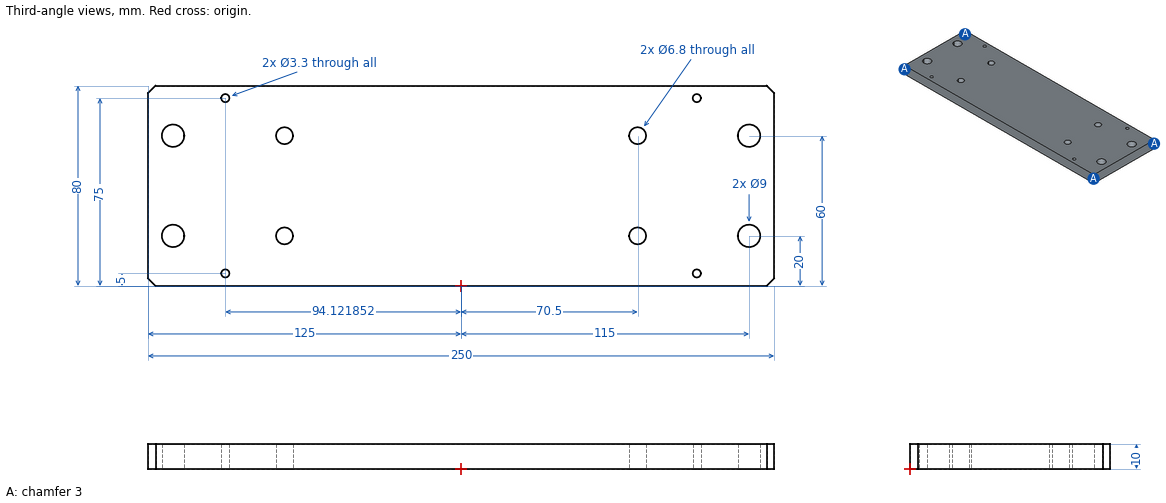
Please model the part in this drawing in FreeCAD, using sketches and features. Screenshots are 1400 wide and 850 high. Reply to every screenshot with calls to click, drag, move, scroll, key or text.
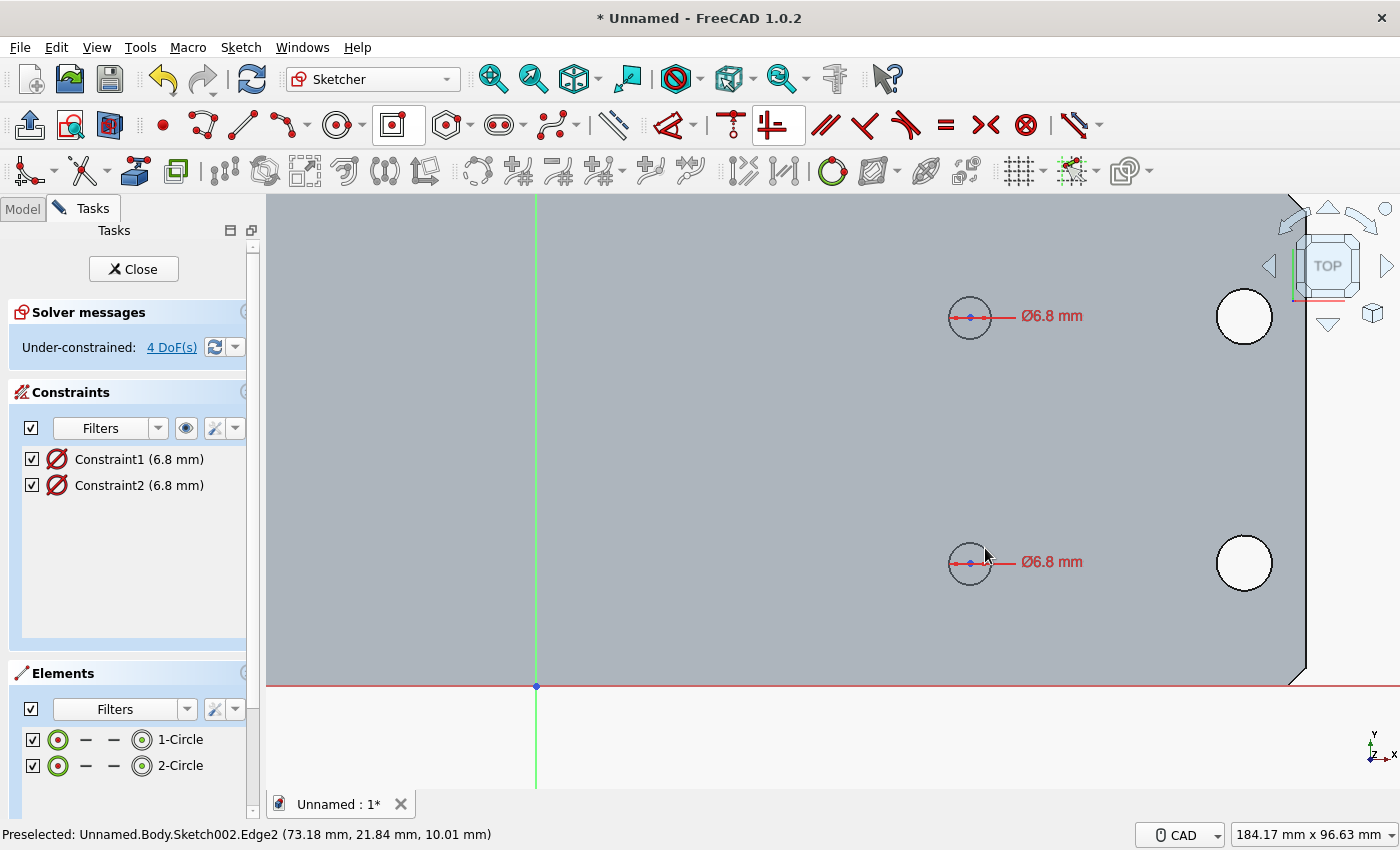
click(970, 318)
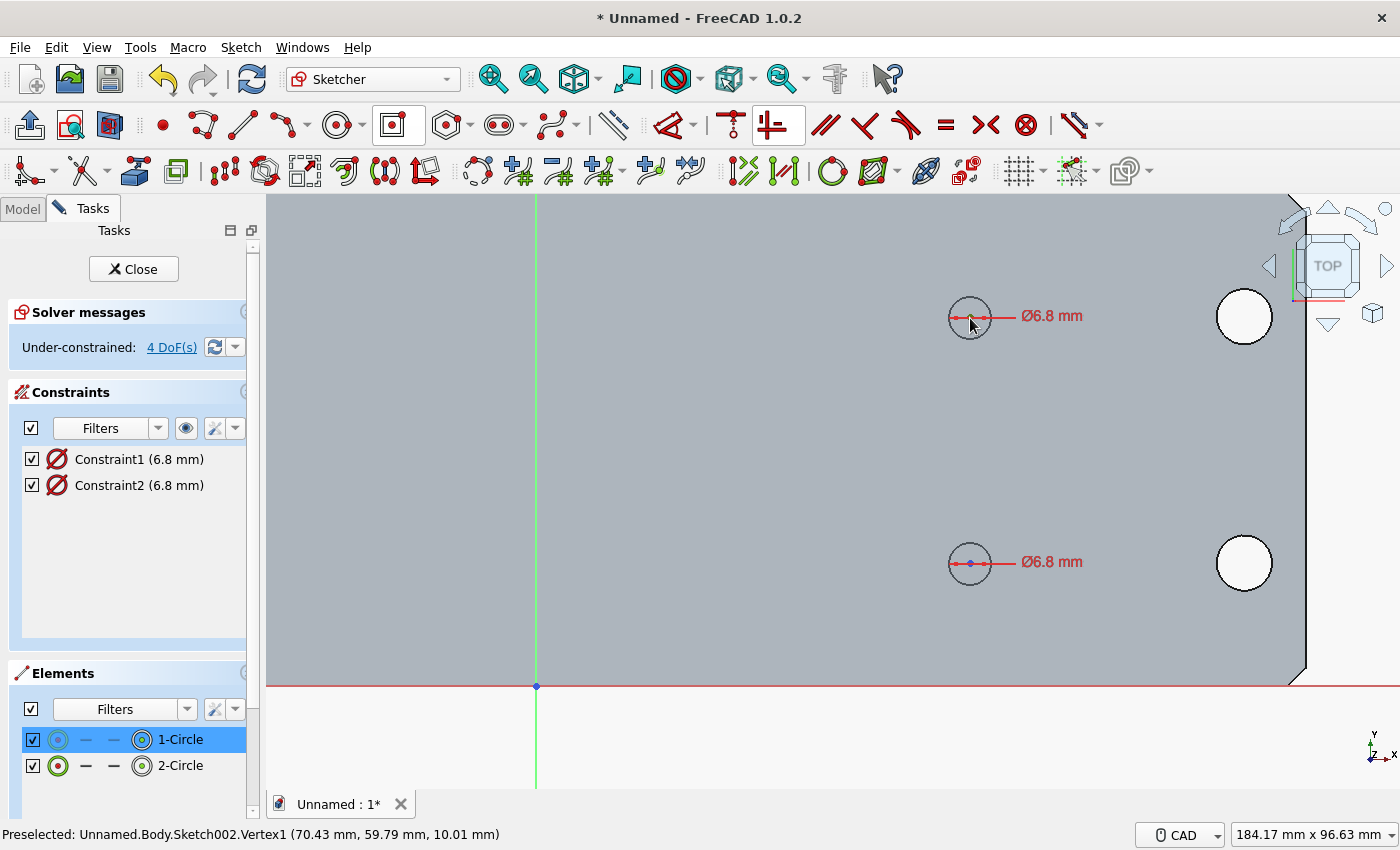
click(970, 564)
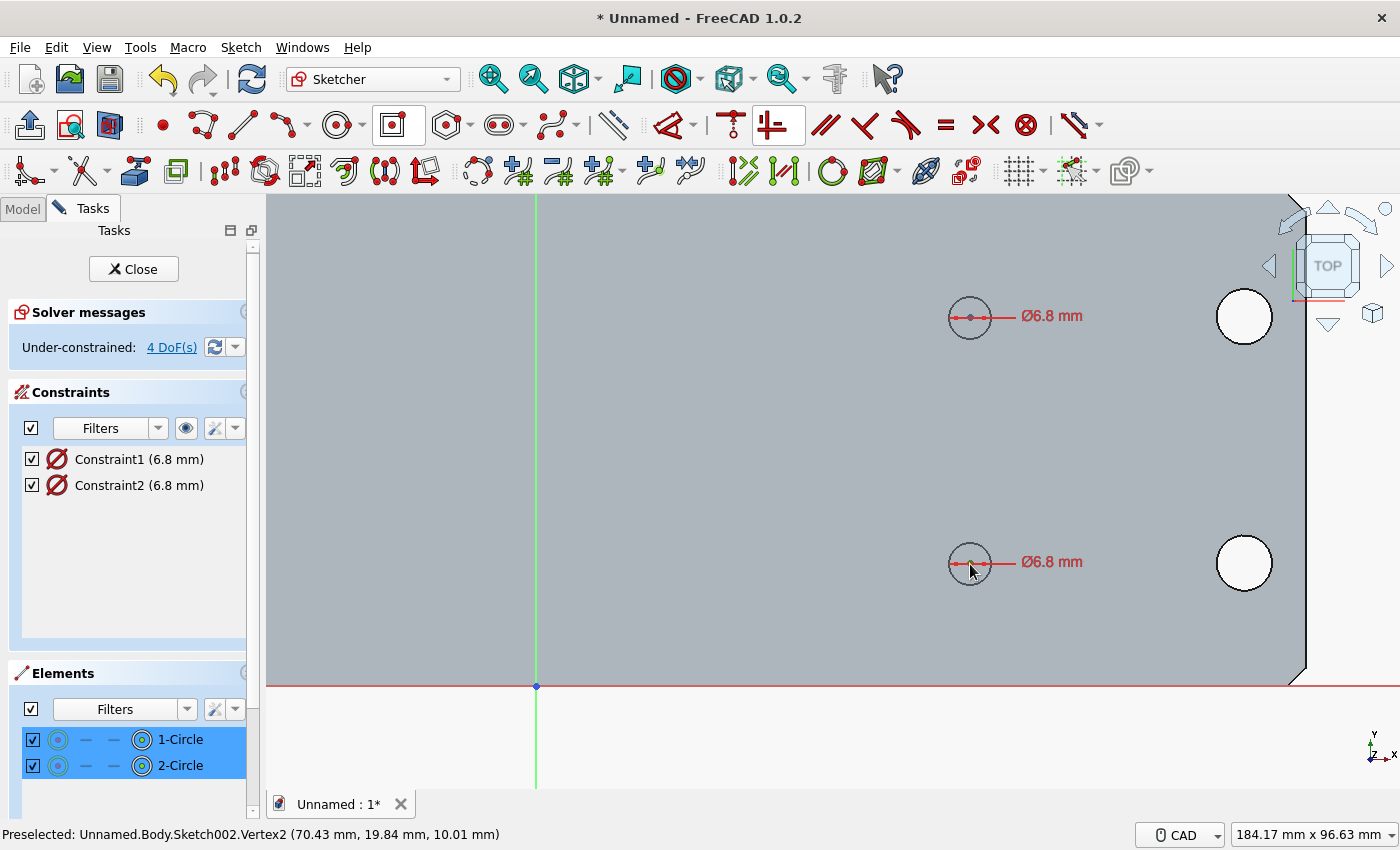
click(800, 126)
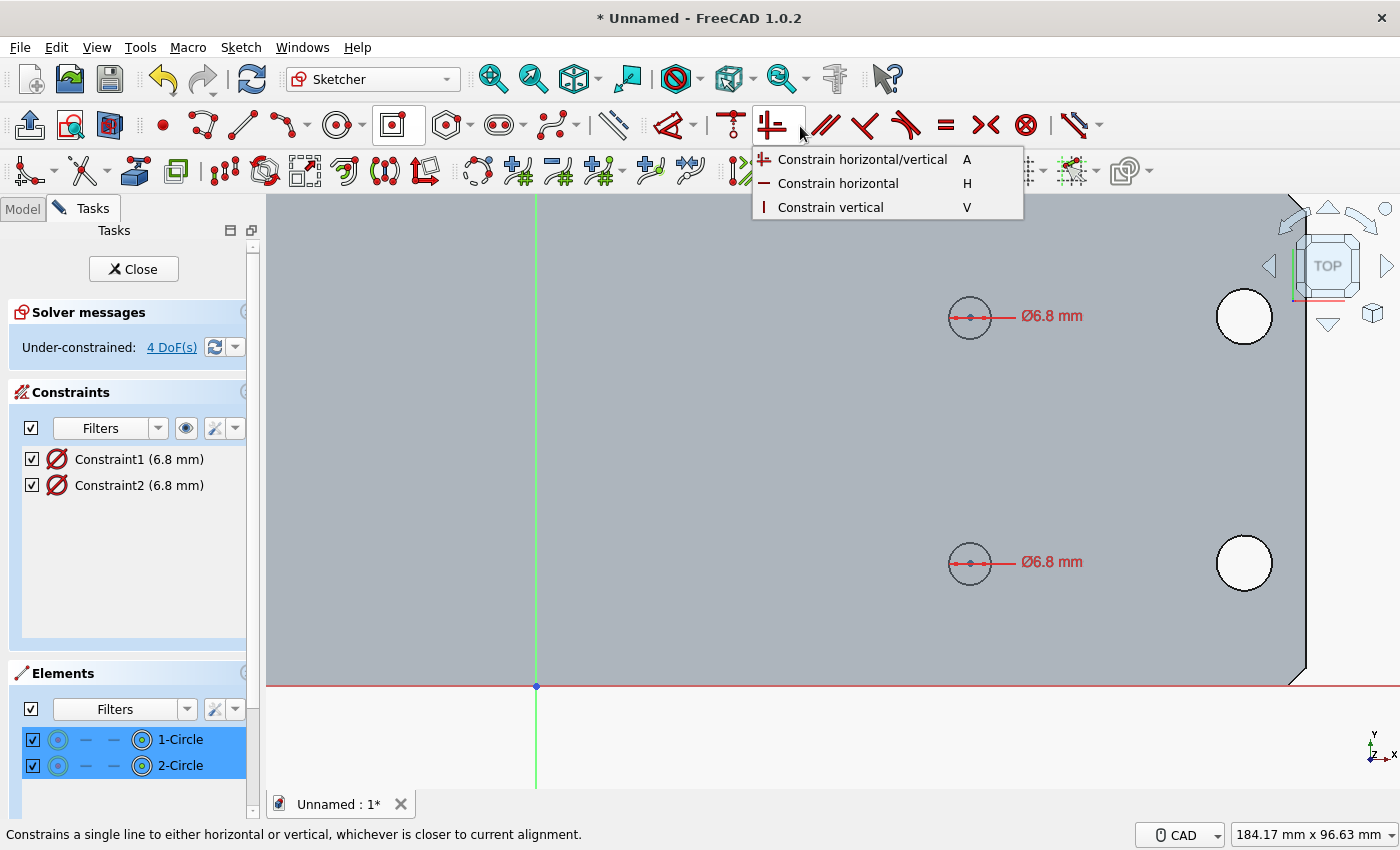
click(888, 207)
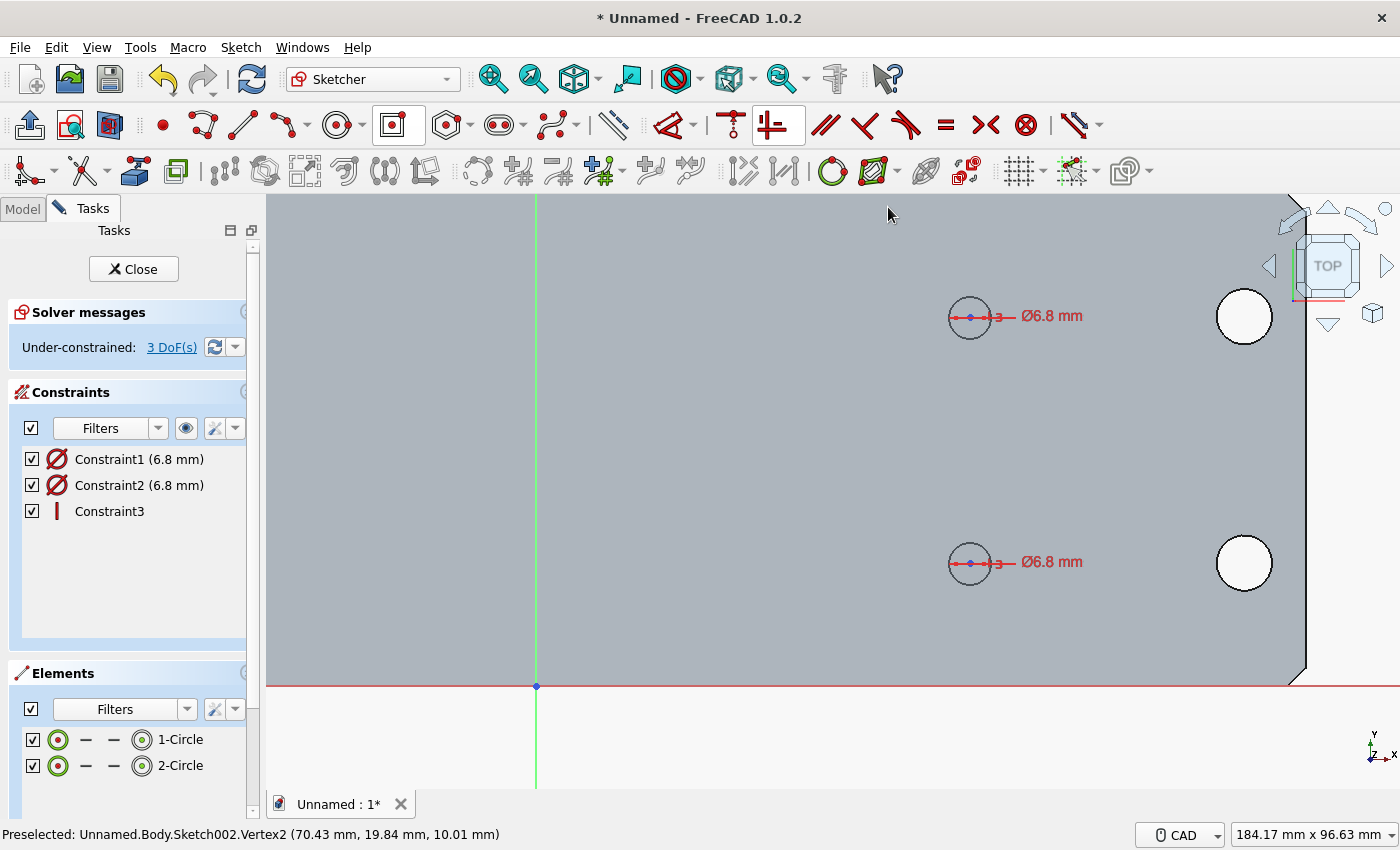
click(668, 126)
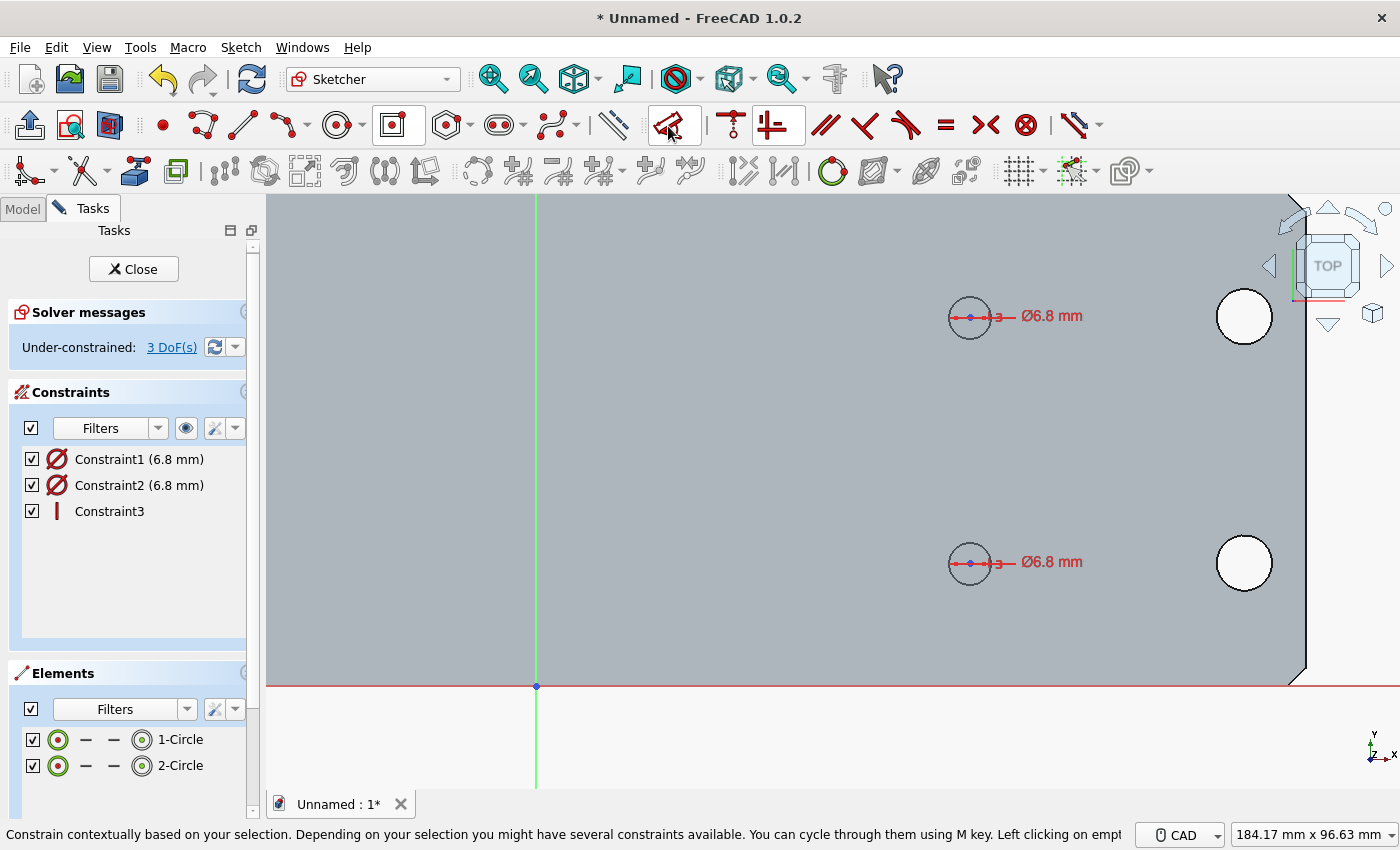
click(970, 318)
click(502, 502)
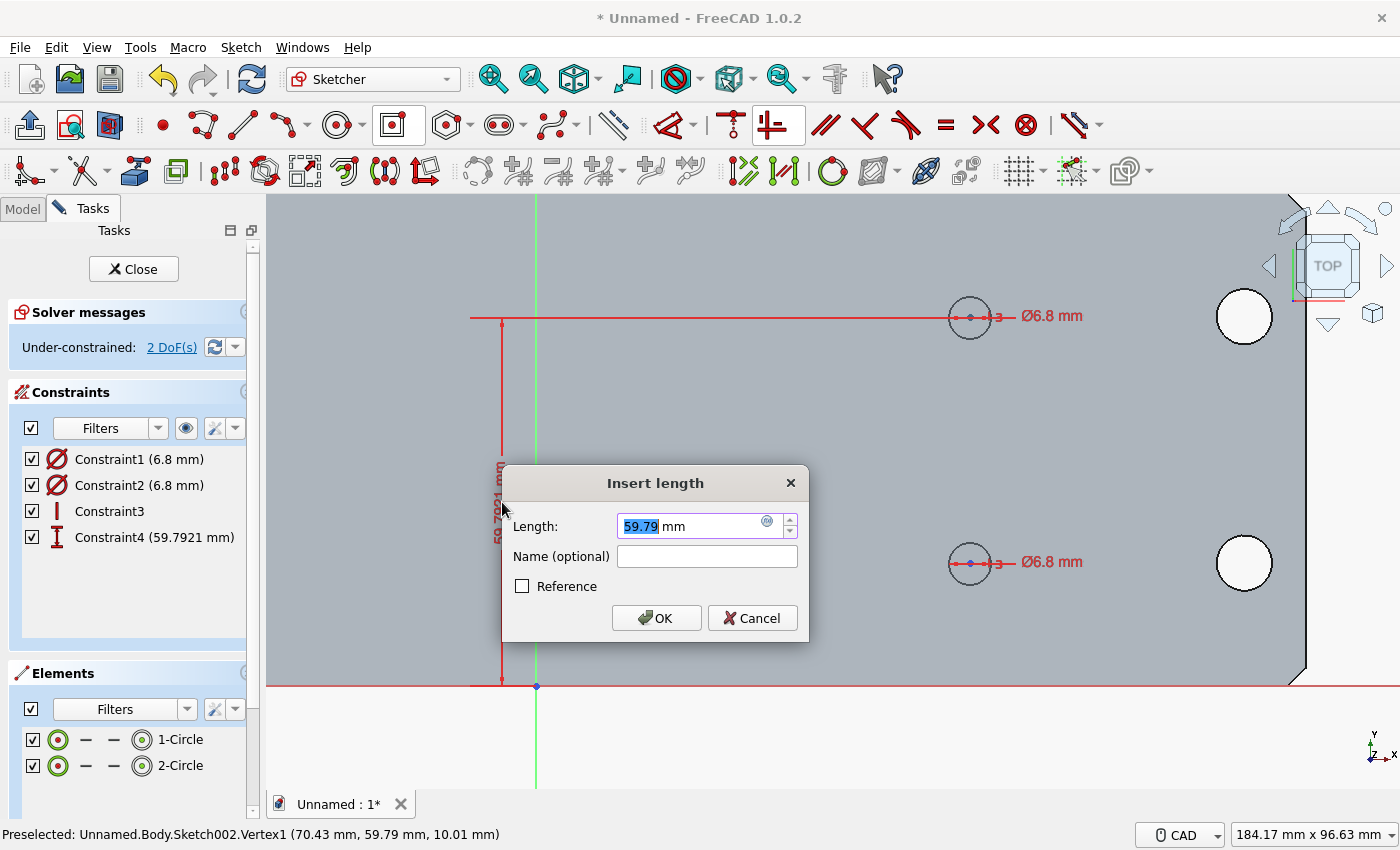
text(60)
key(Return)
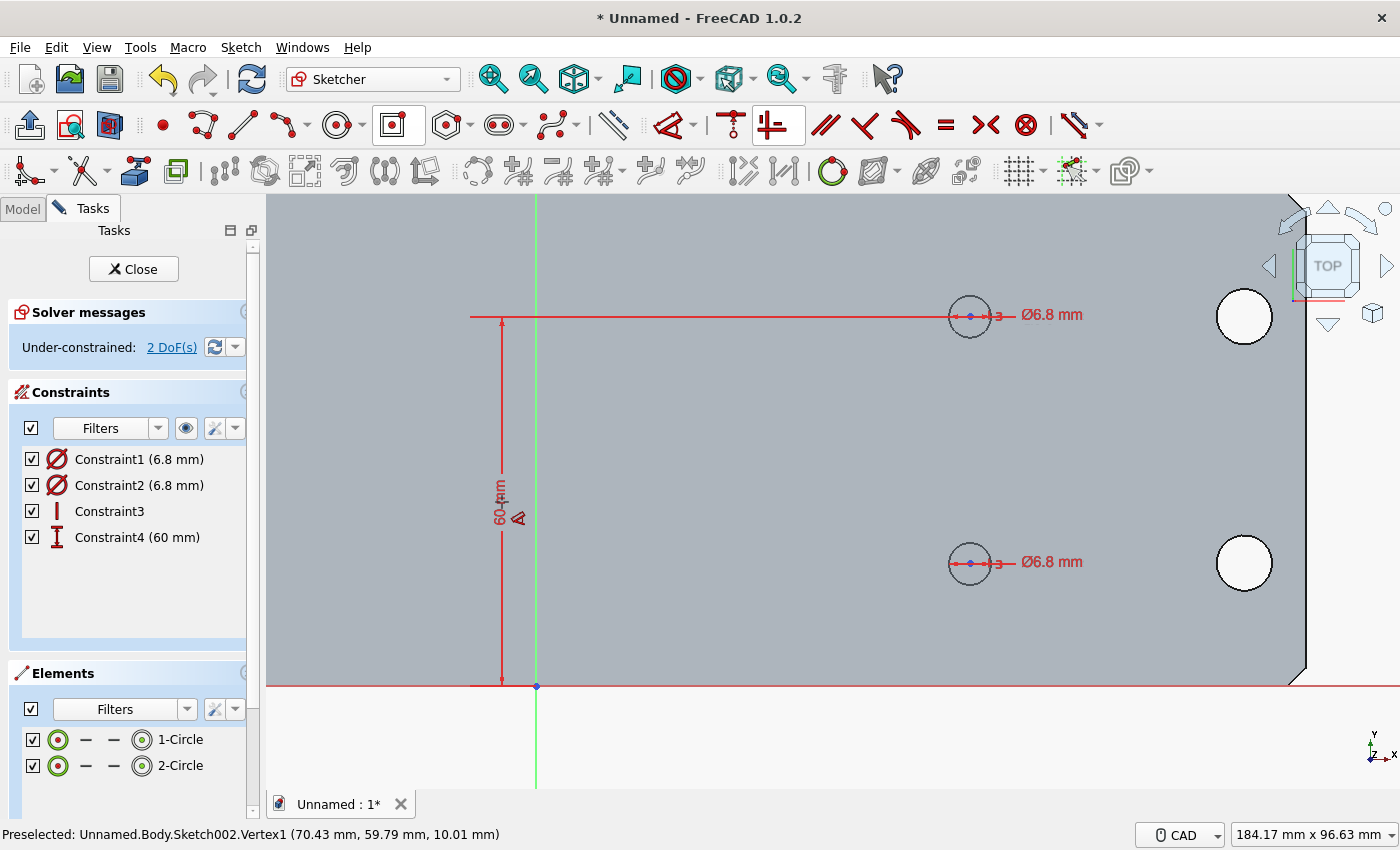
click(970, 564)
click(502, 625)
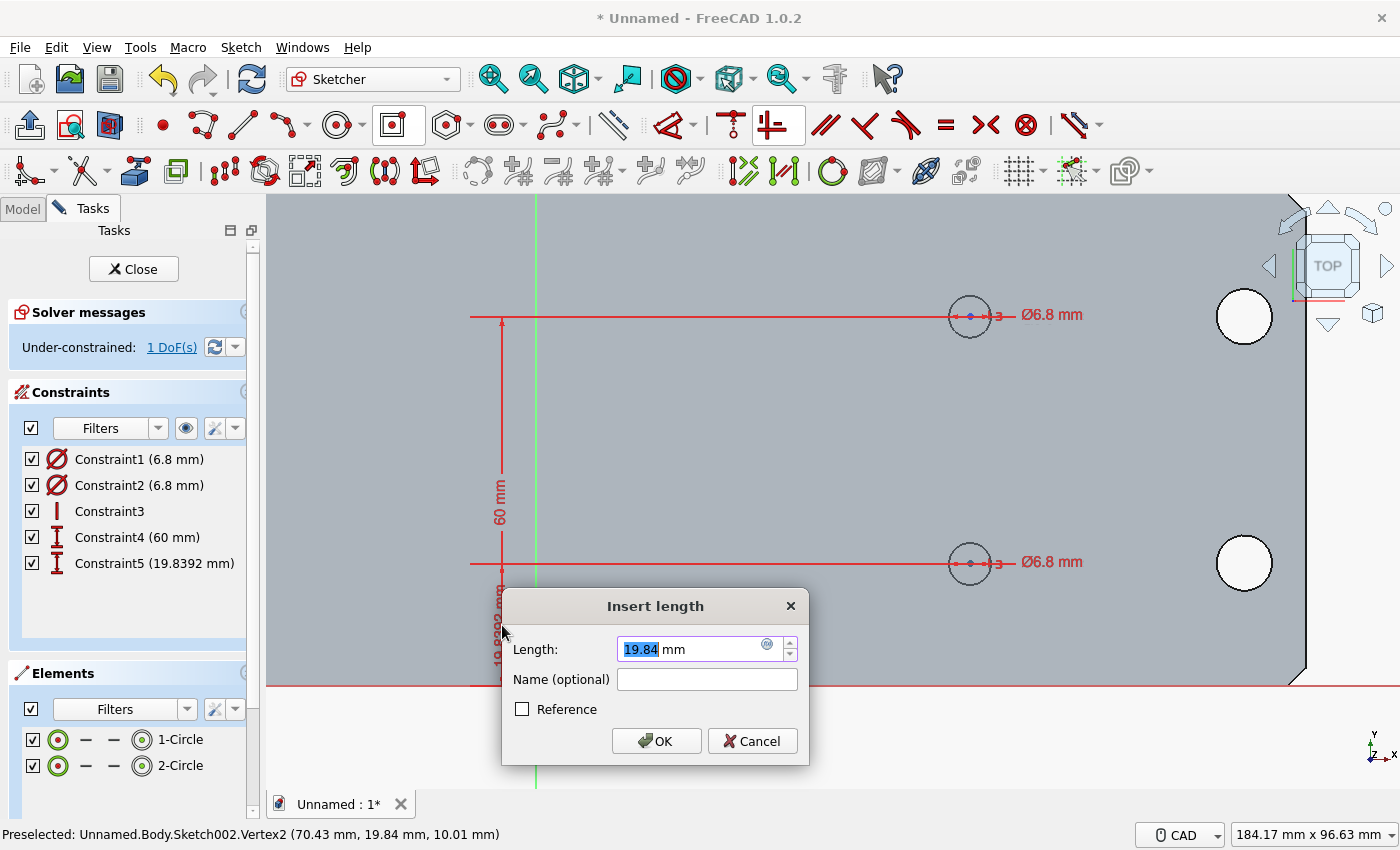
text(20)
key(Return)